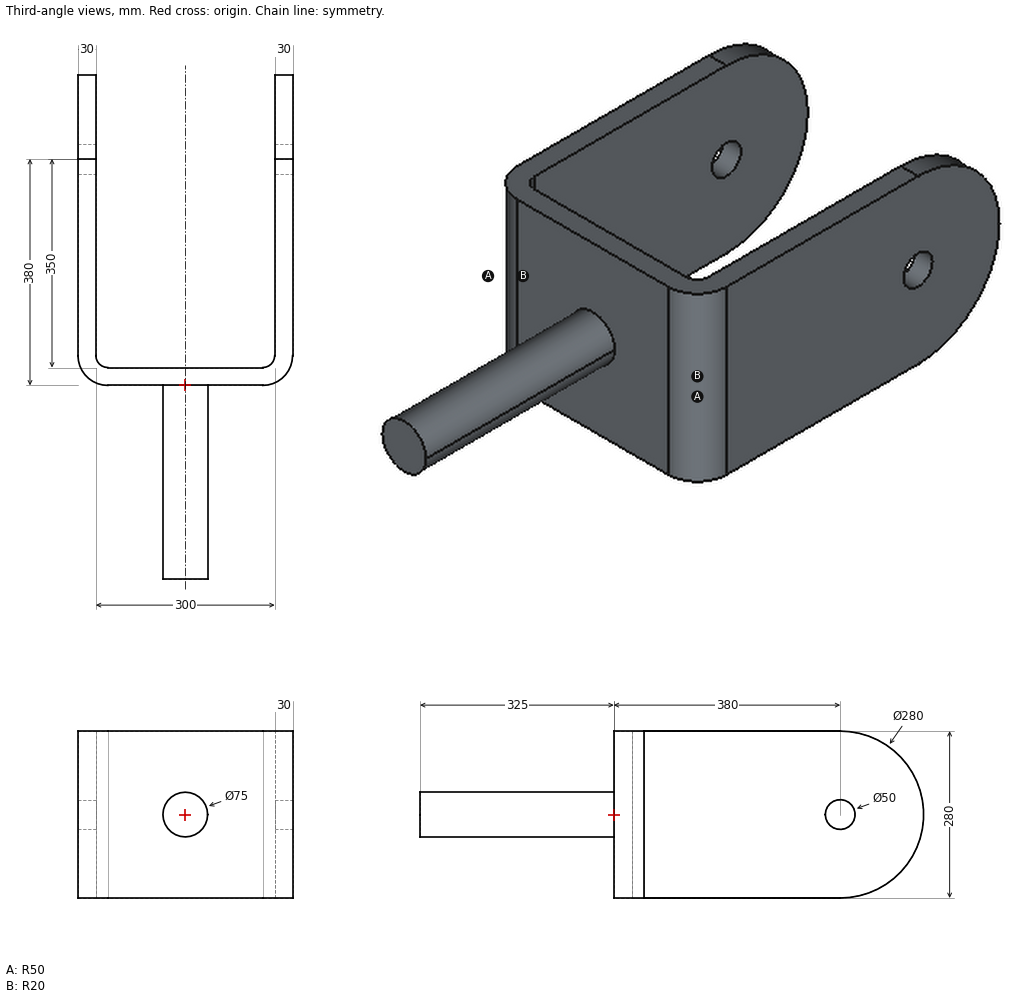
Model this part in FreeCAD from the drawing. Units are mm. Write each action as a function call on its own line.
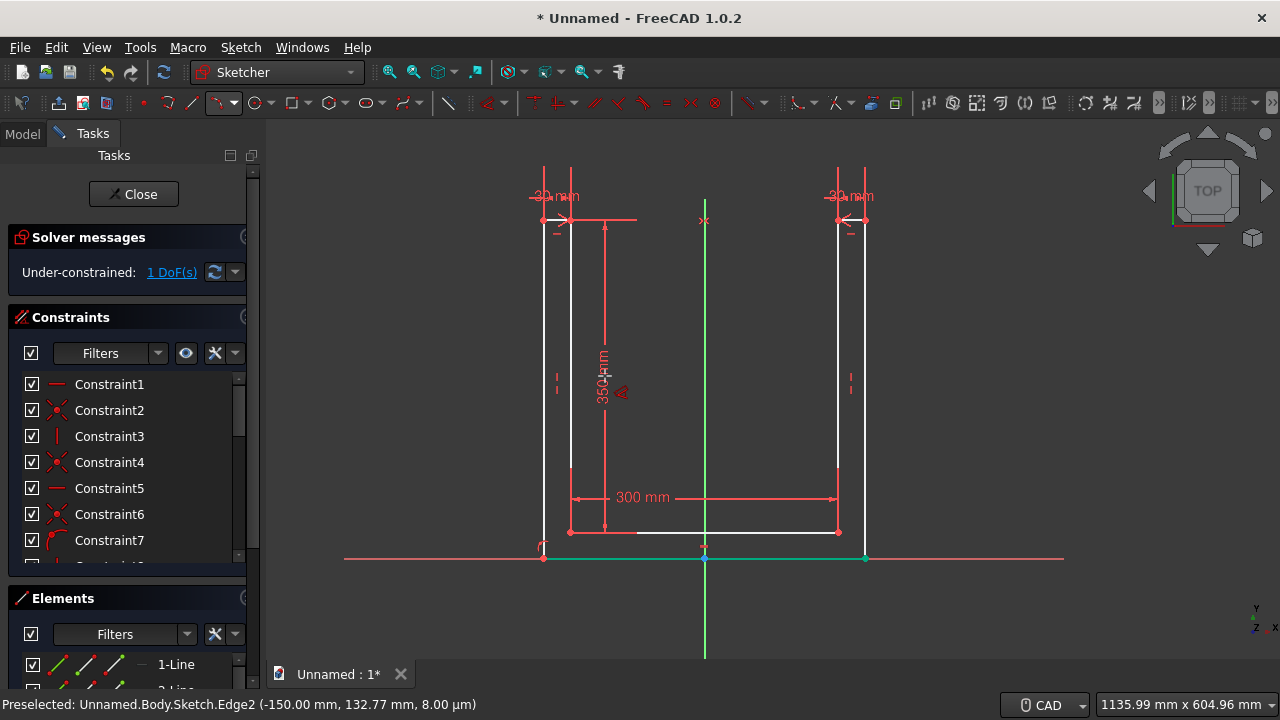
click(544, 322)
click(510, 389)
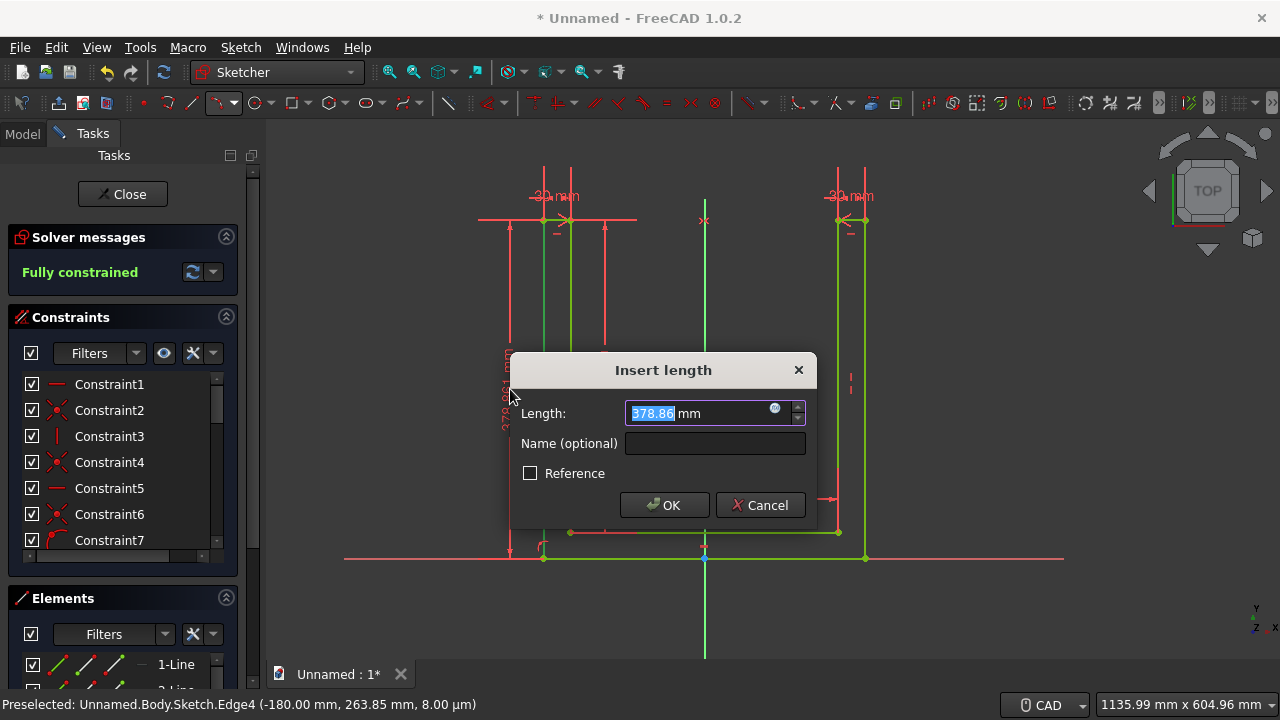
text(380)
key(Return)
key(Escape)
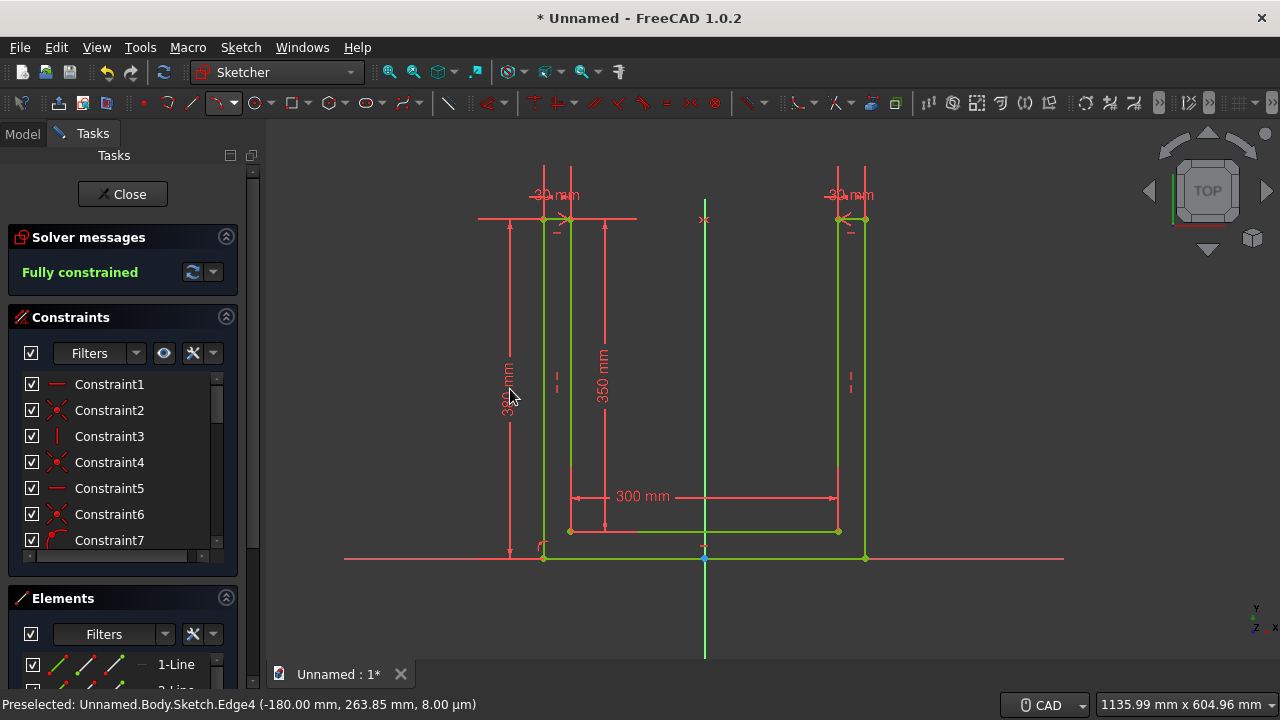
click(123, 194)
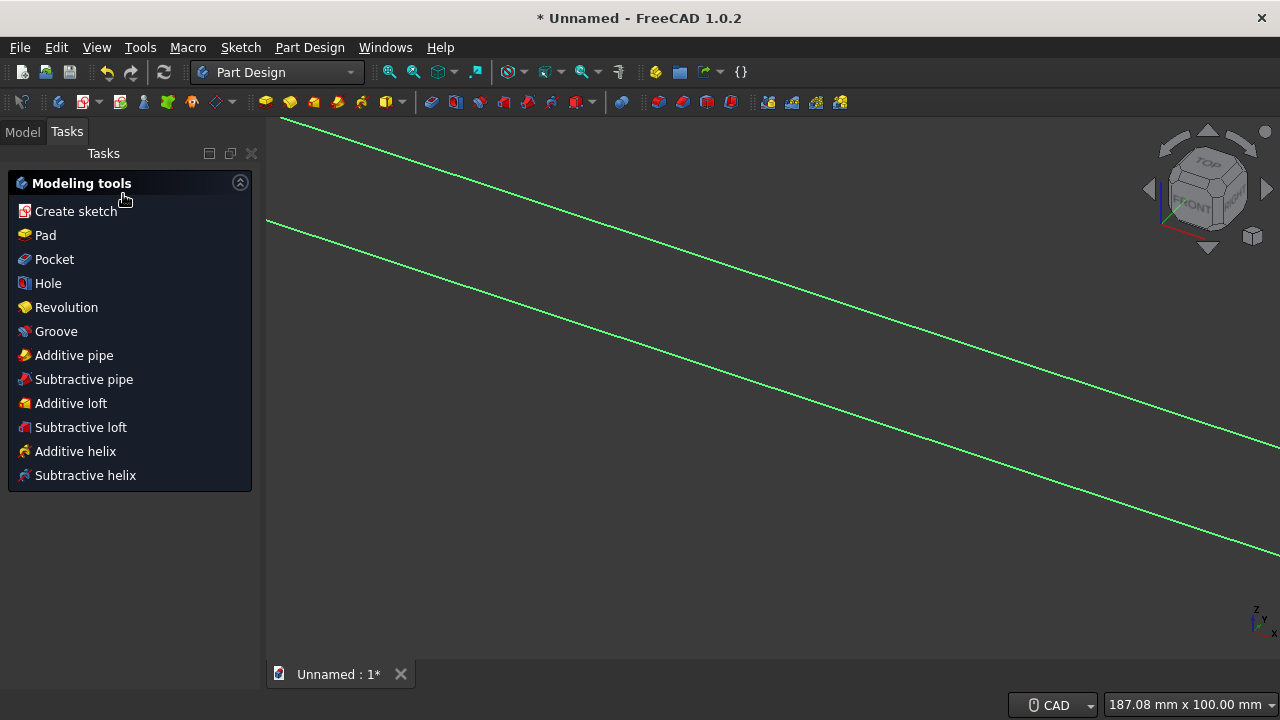
click(266, 102)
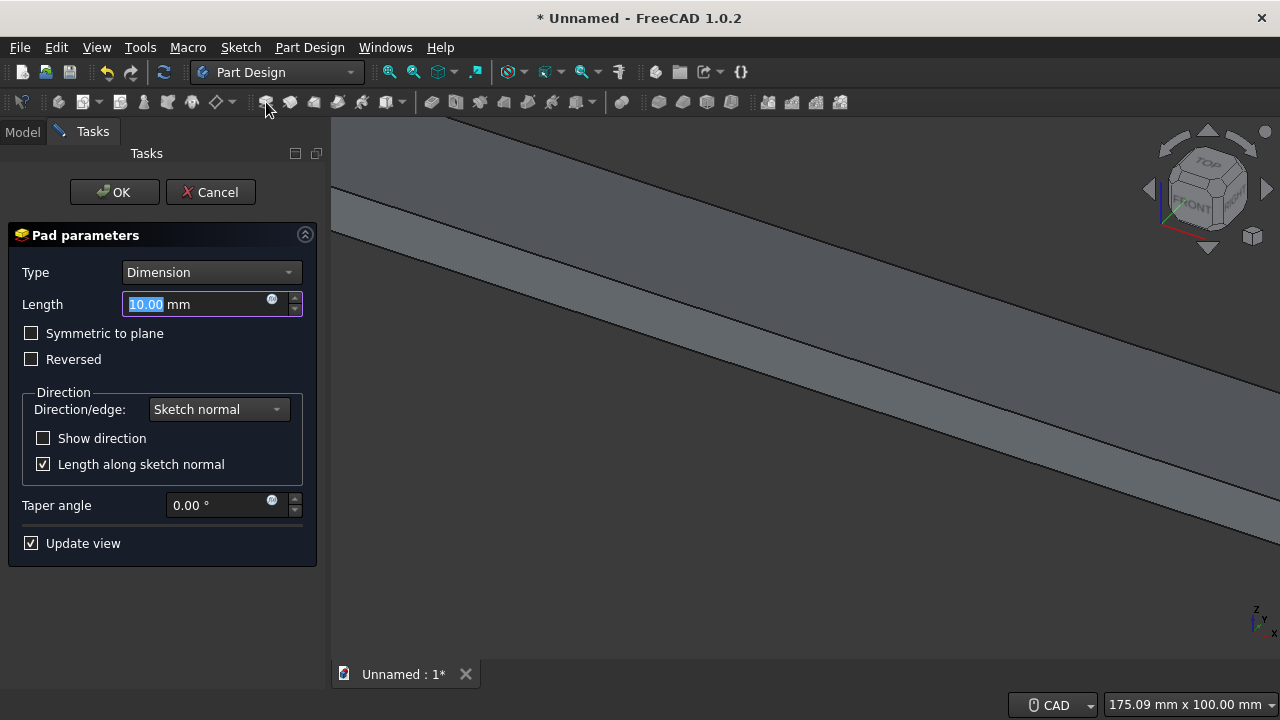
text(280)
key(Tab)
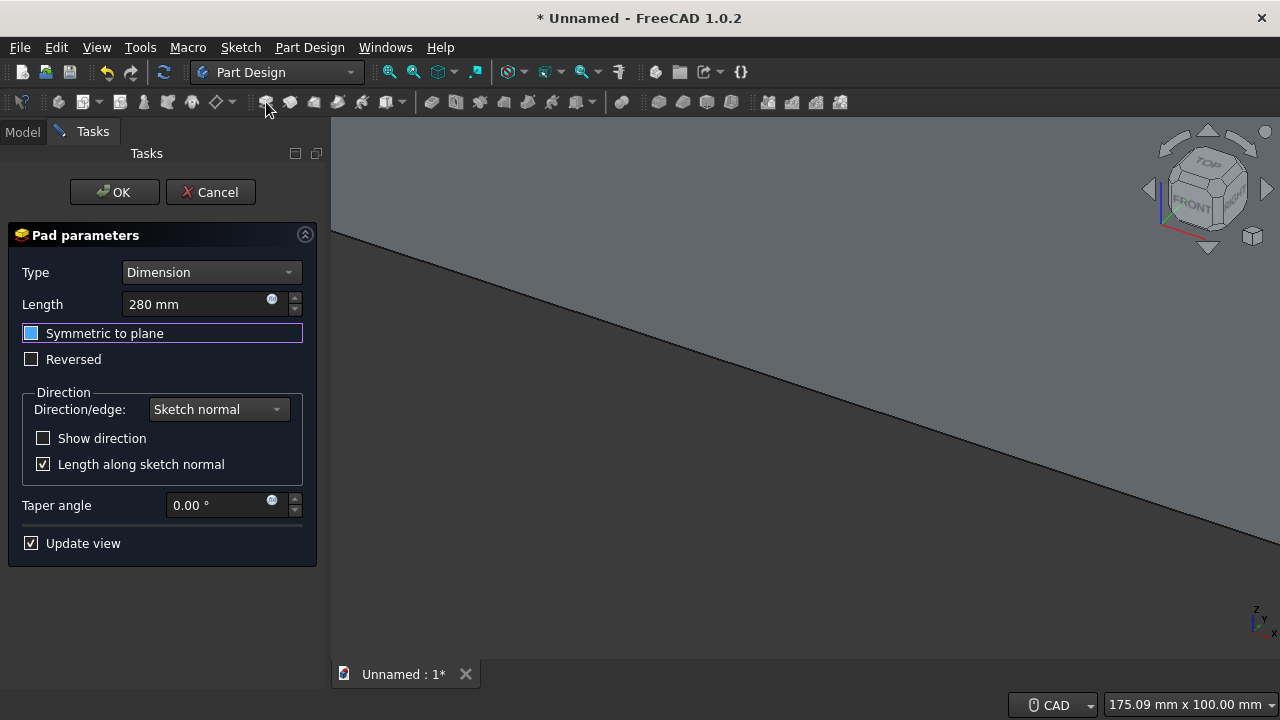
click(30, 333)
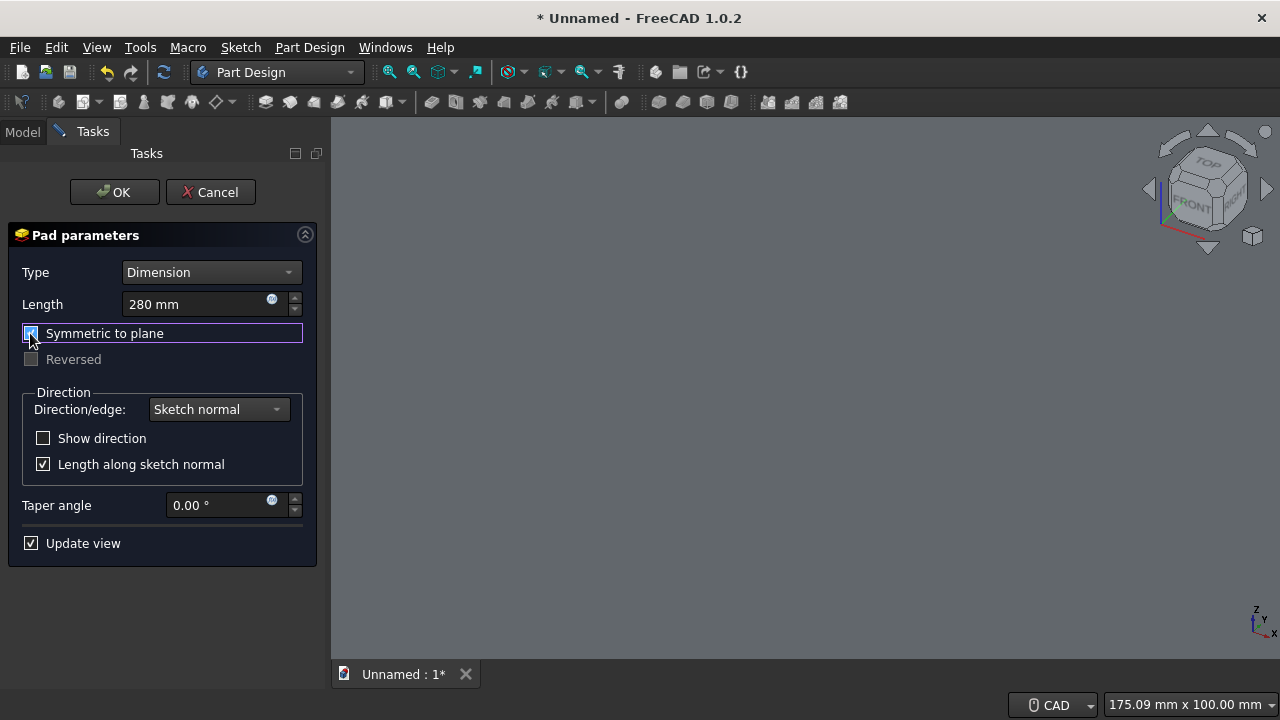
click(115, 192)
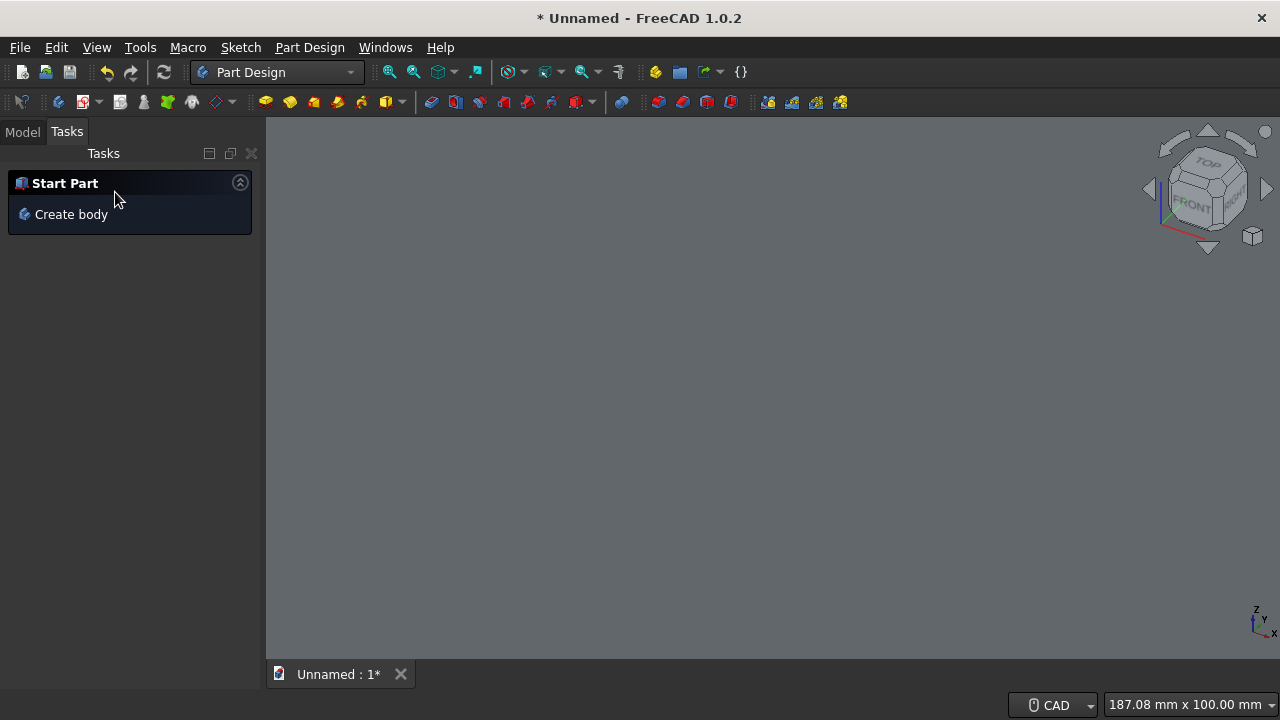
click(390, 72)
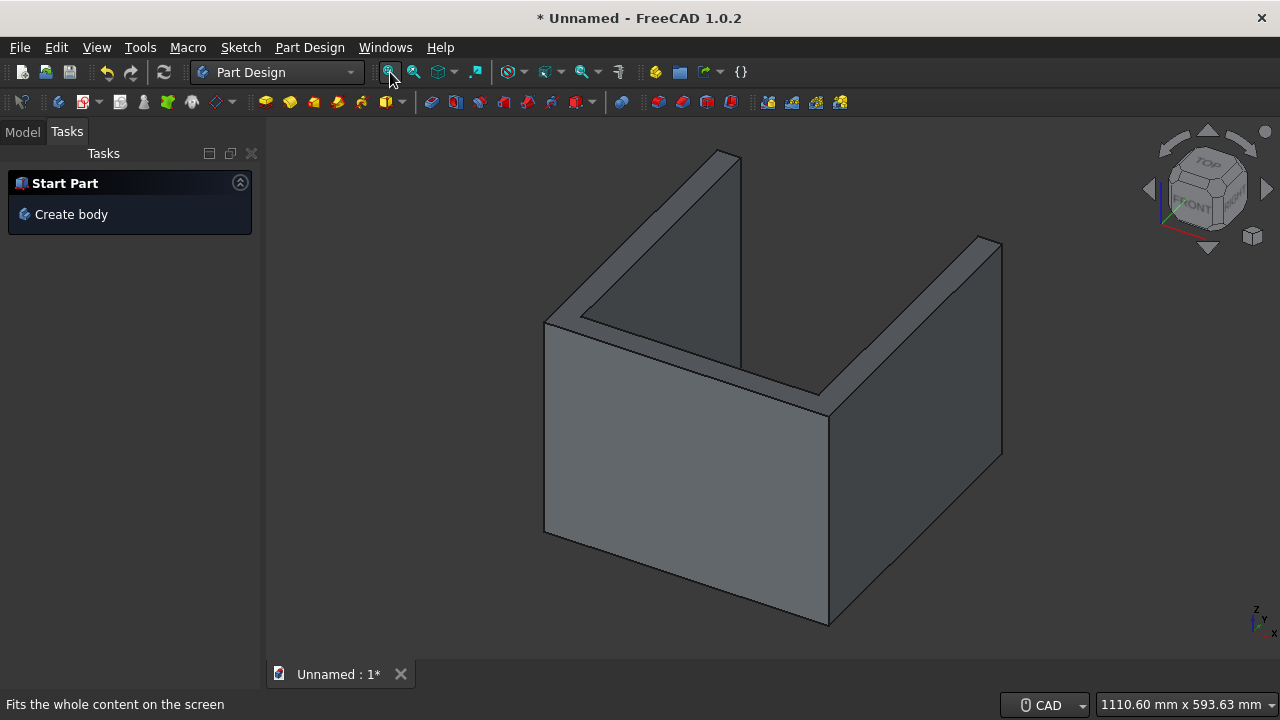
click(84, 102)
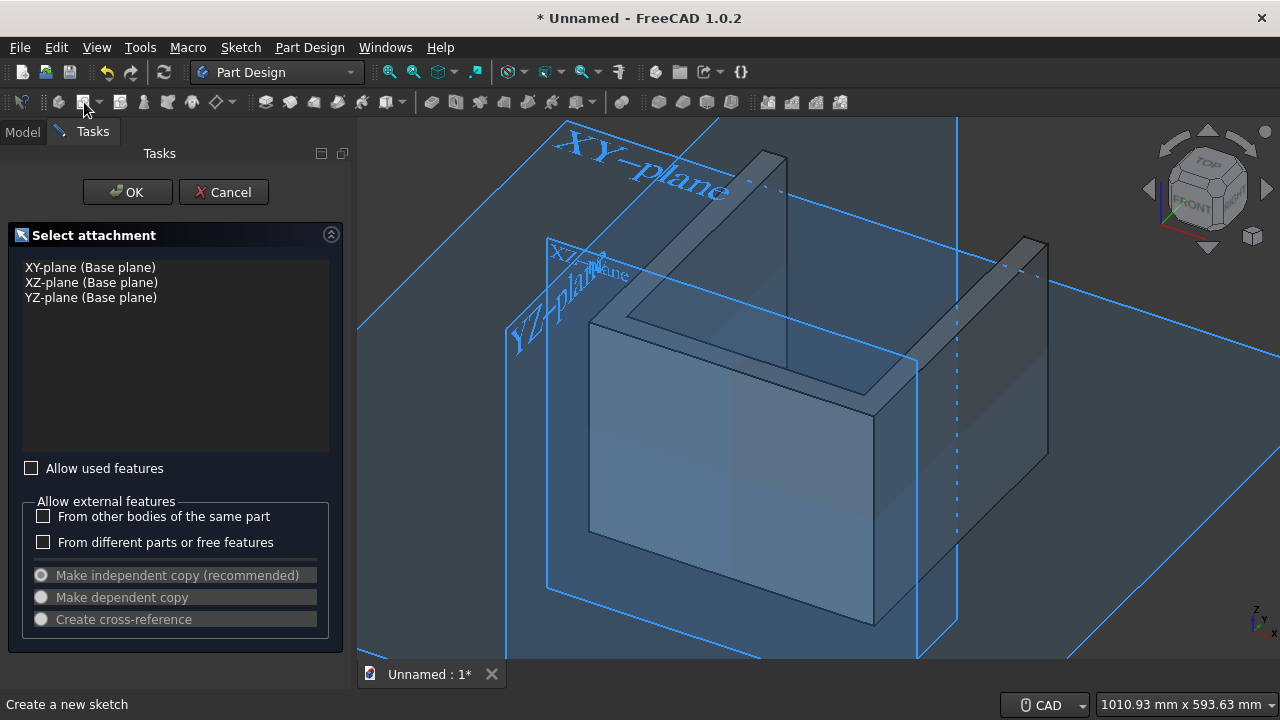
click(82, 282)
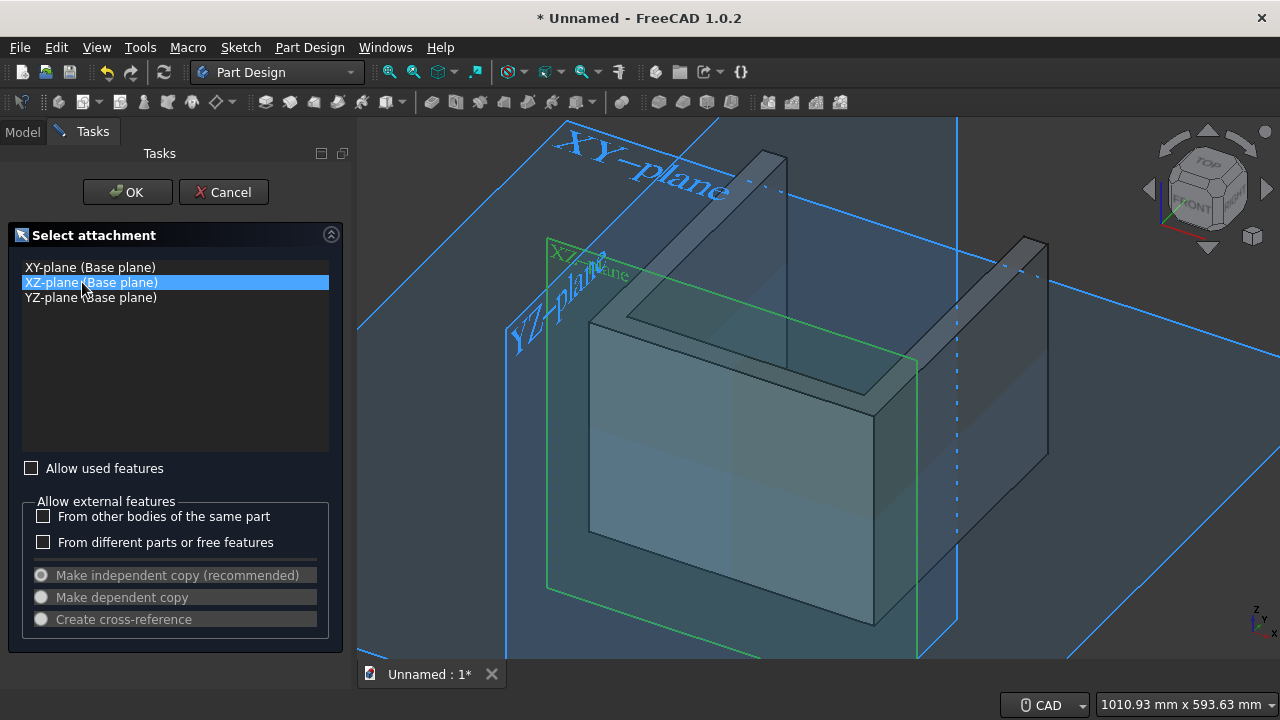
click(128, 192)